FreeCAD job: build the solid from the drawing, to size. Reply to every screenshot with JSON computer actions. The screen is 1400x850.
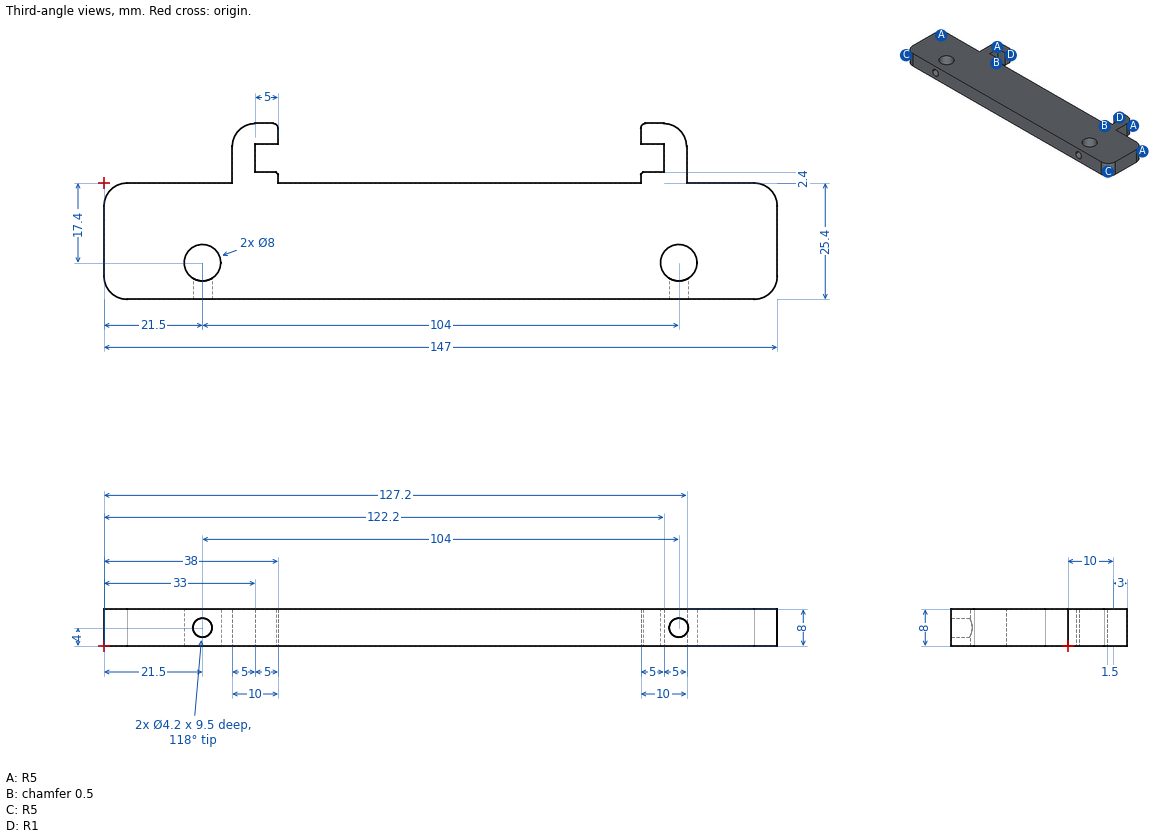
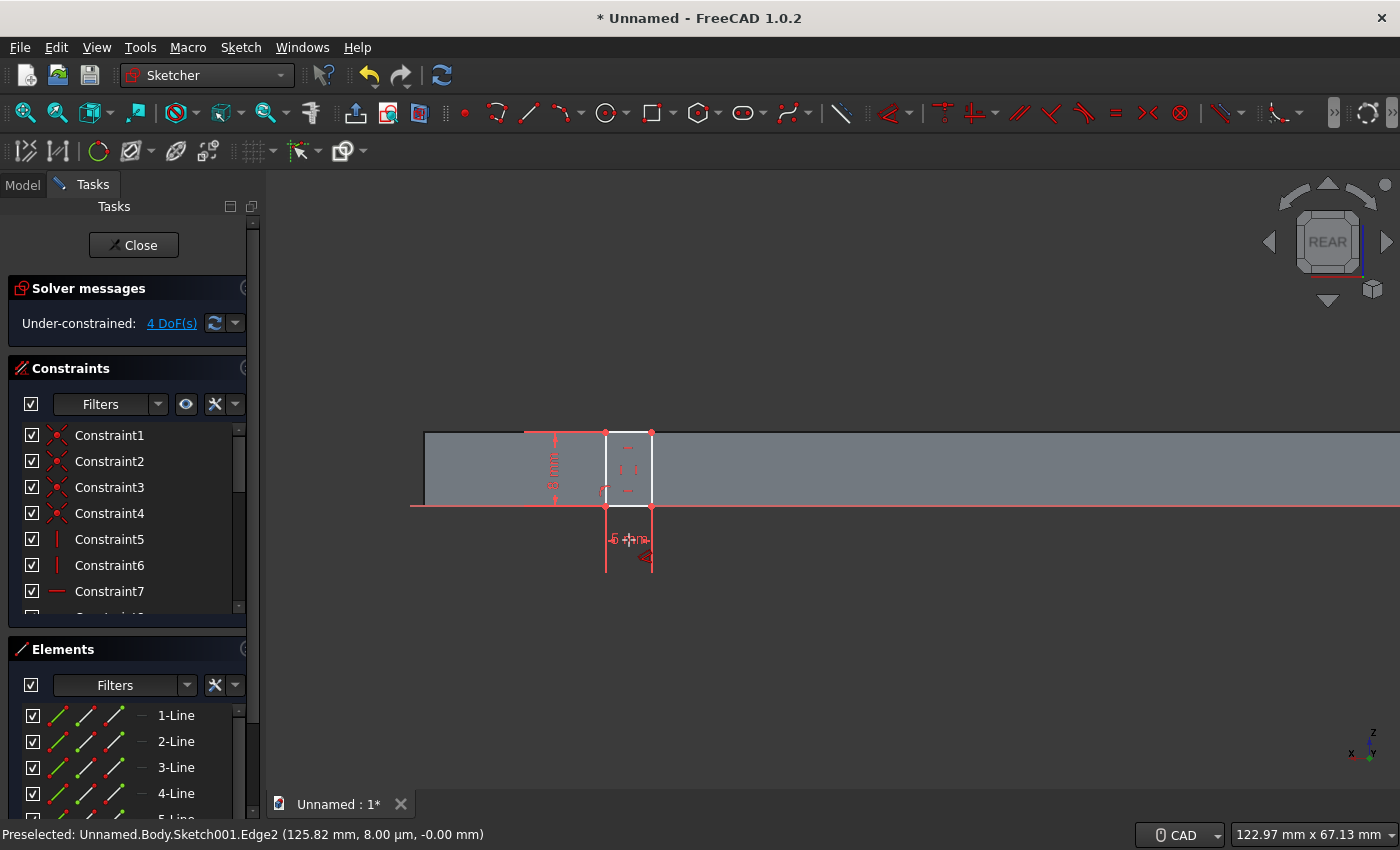
{"action": "scroll", "coordinate": [294, 492], "scroll_direction": "down", "scroll_amount": 3}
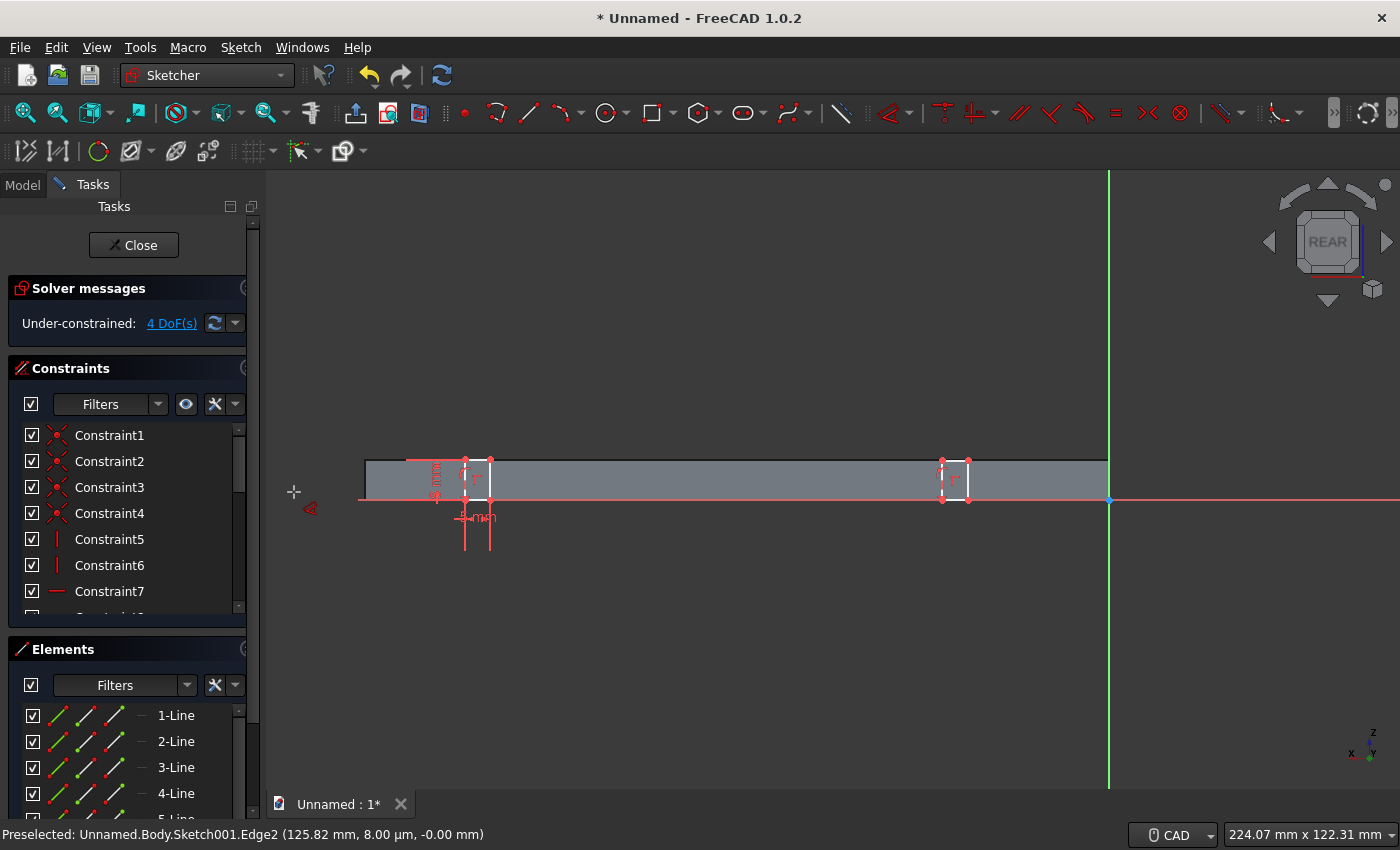
{"action": "left_click", "coordinate": [942, 473]}
{"action": "left_click", "coordinate": [908, 480]}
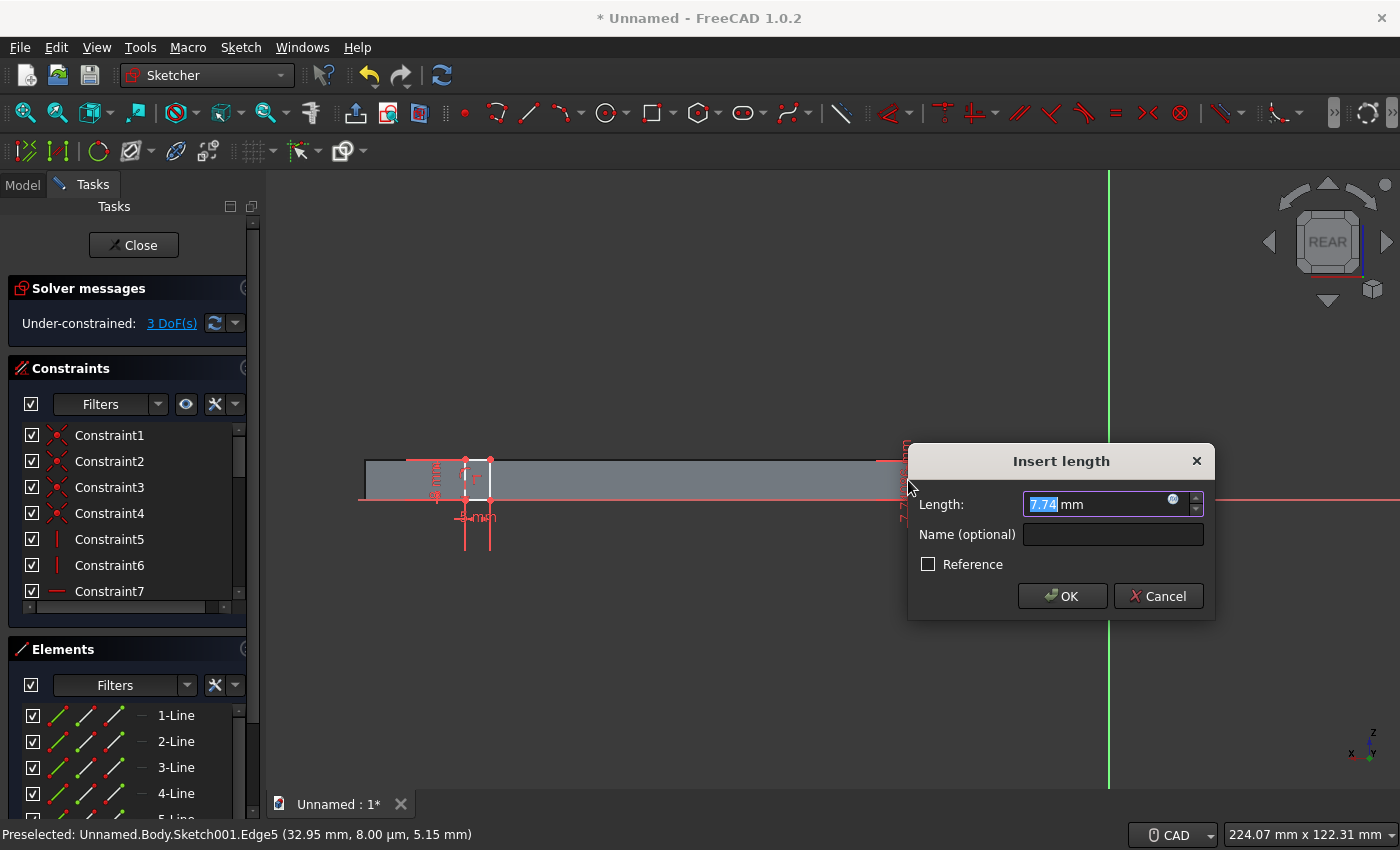
{"action": "type", "text": "8"}
{"action": "key", "text": "Return"}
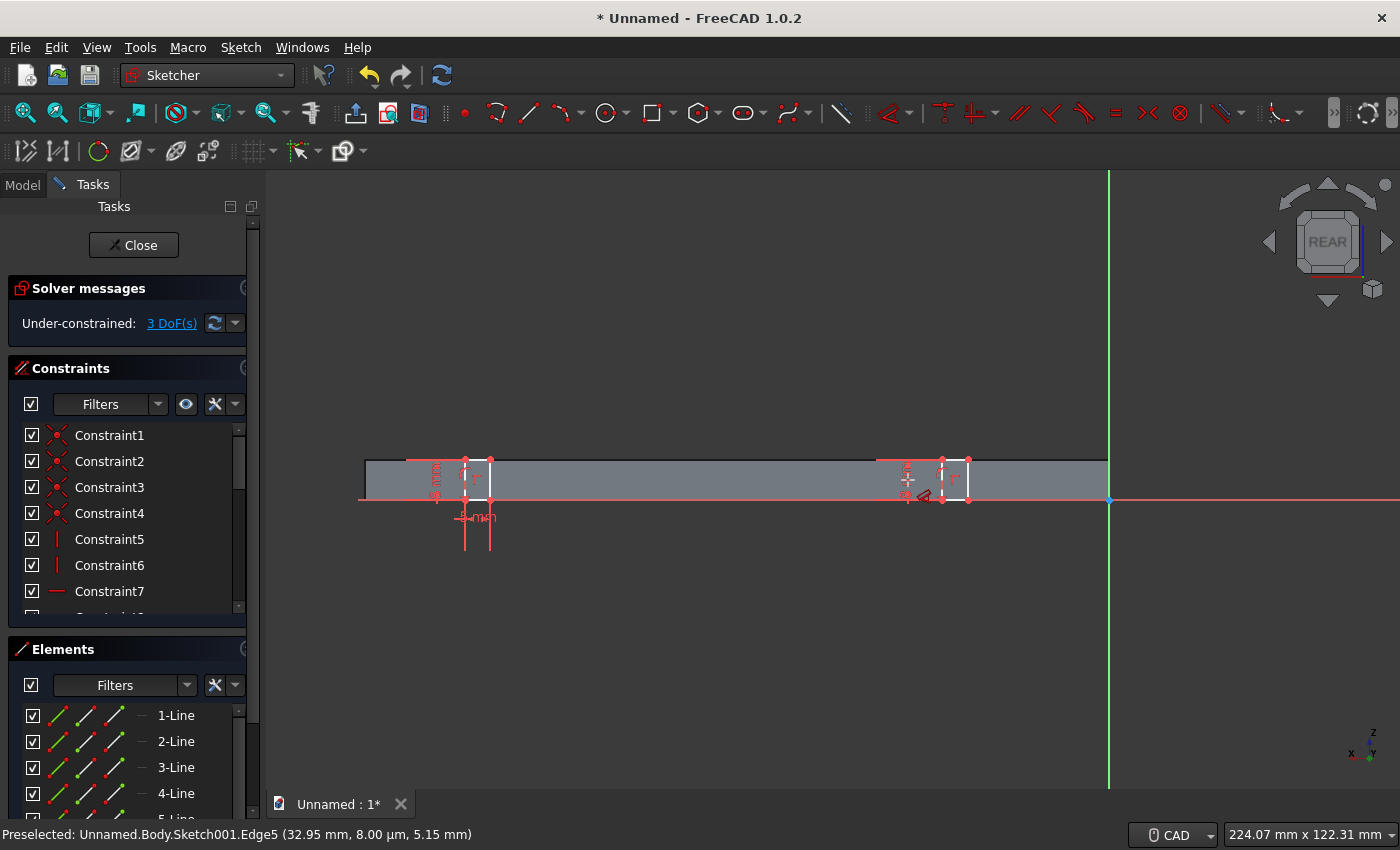
{"action": "scroll", "coordinate": [953, 500], "scroll_direction": "up", "scroll_amount": 3}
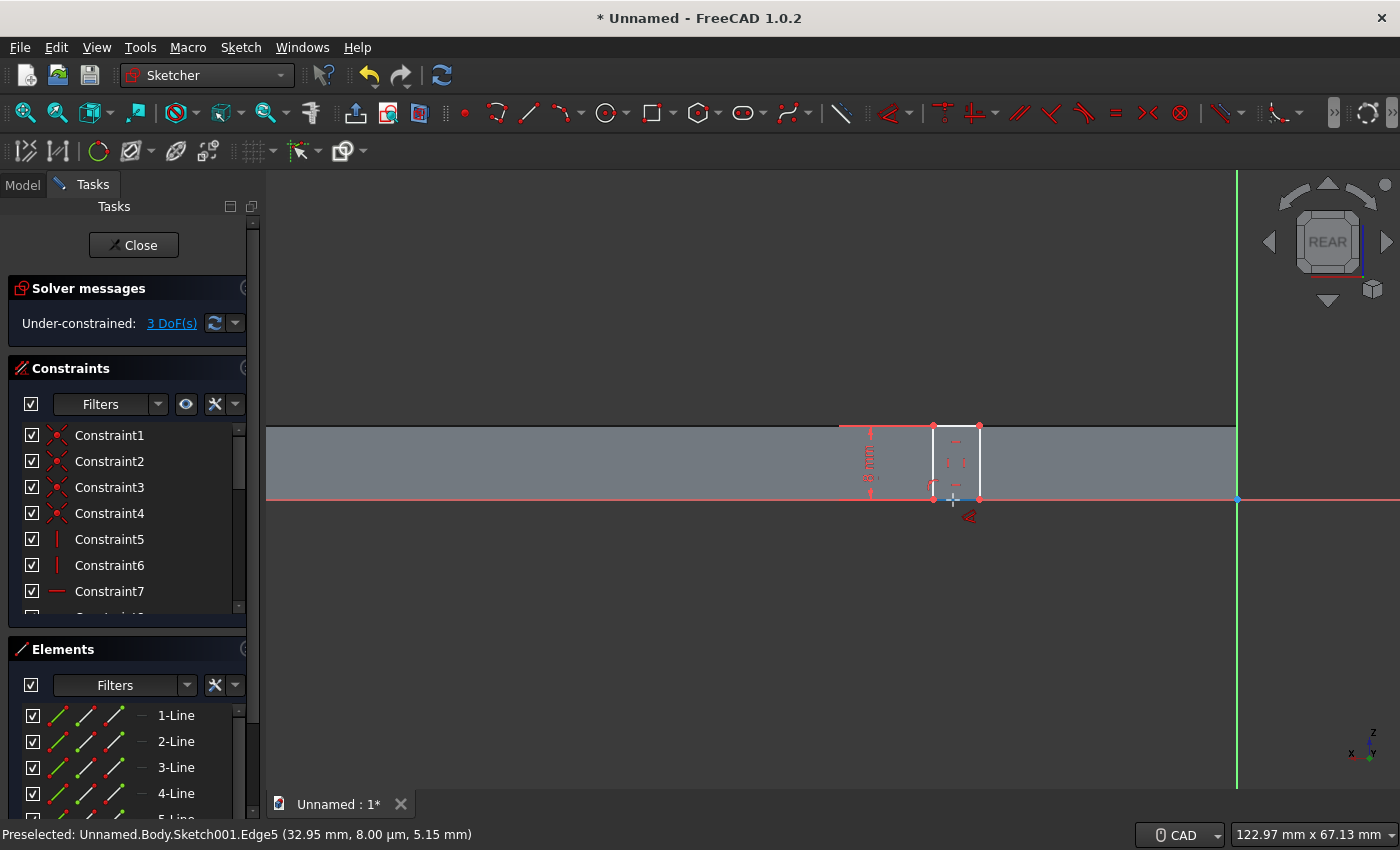
{"action": "left_click", "coordinate": [952, 500]}
{"action": "left_click", "coordinate": [956, 534]}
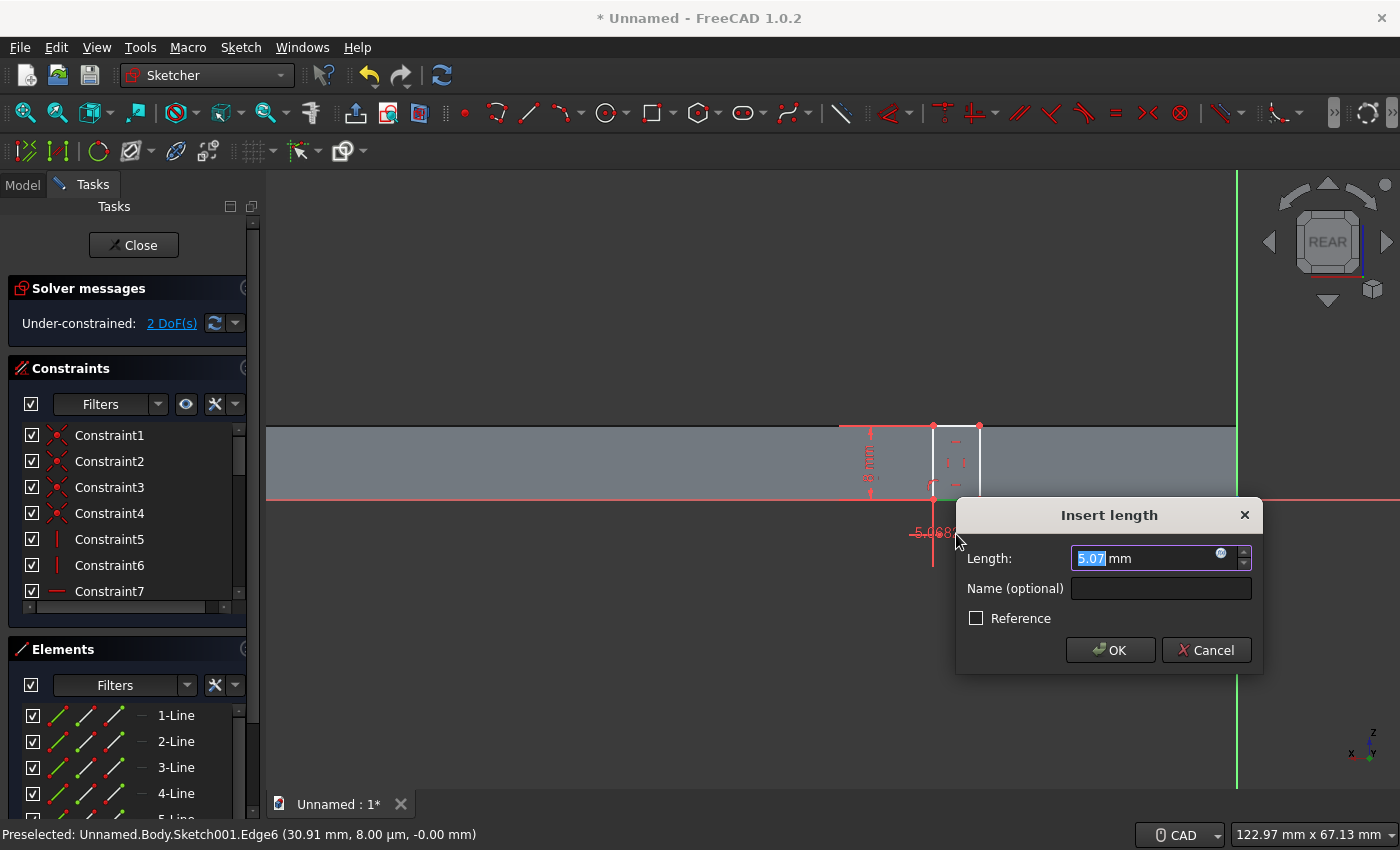
{"action": "type", "text": "5"}
{"action": "key", "text": "Return"}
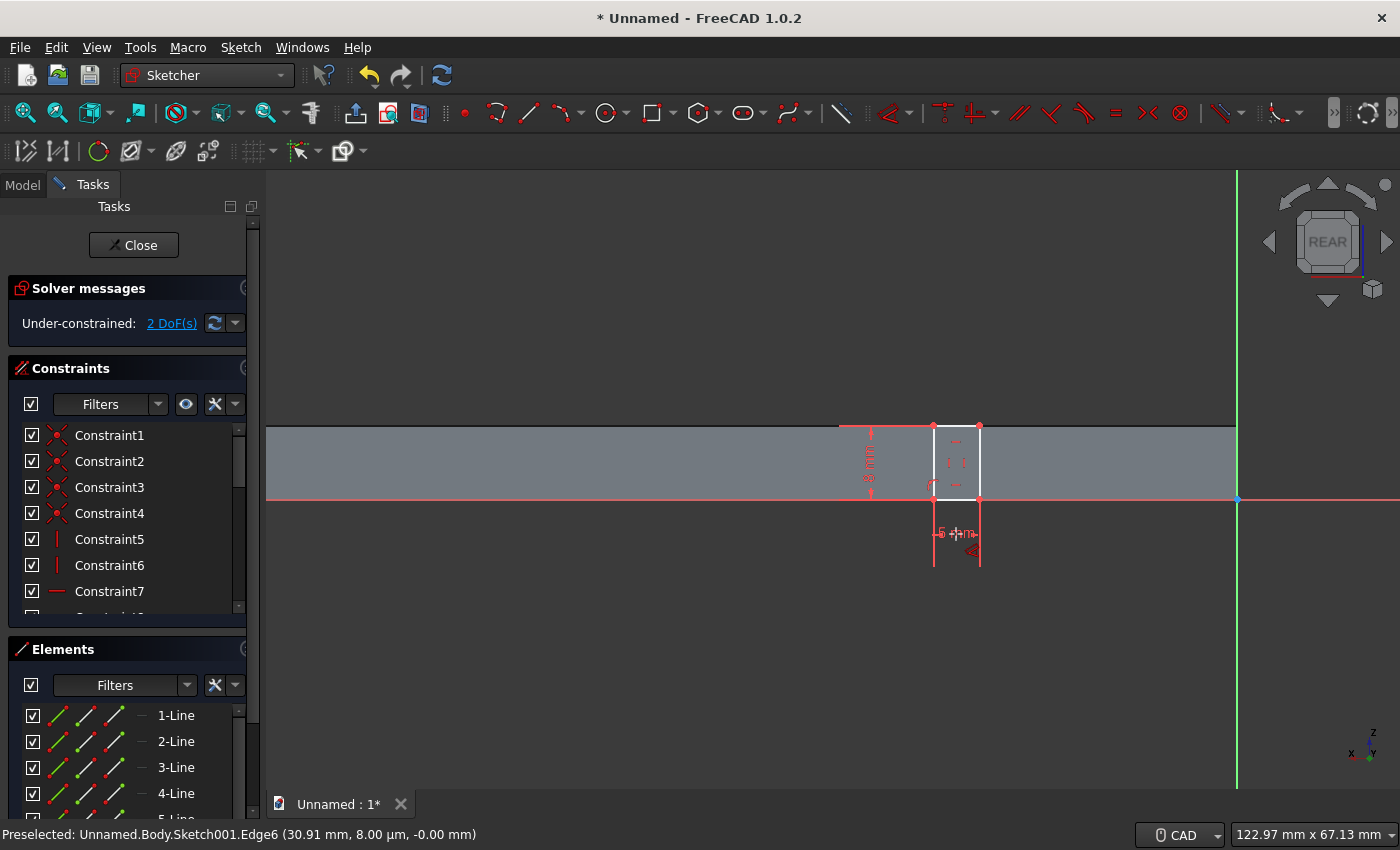
{"action": "left_click", "coordinate": [934, 426]}
{"action": "left_click", "coordinate": [1084, 534]}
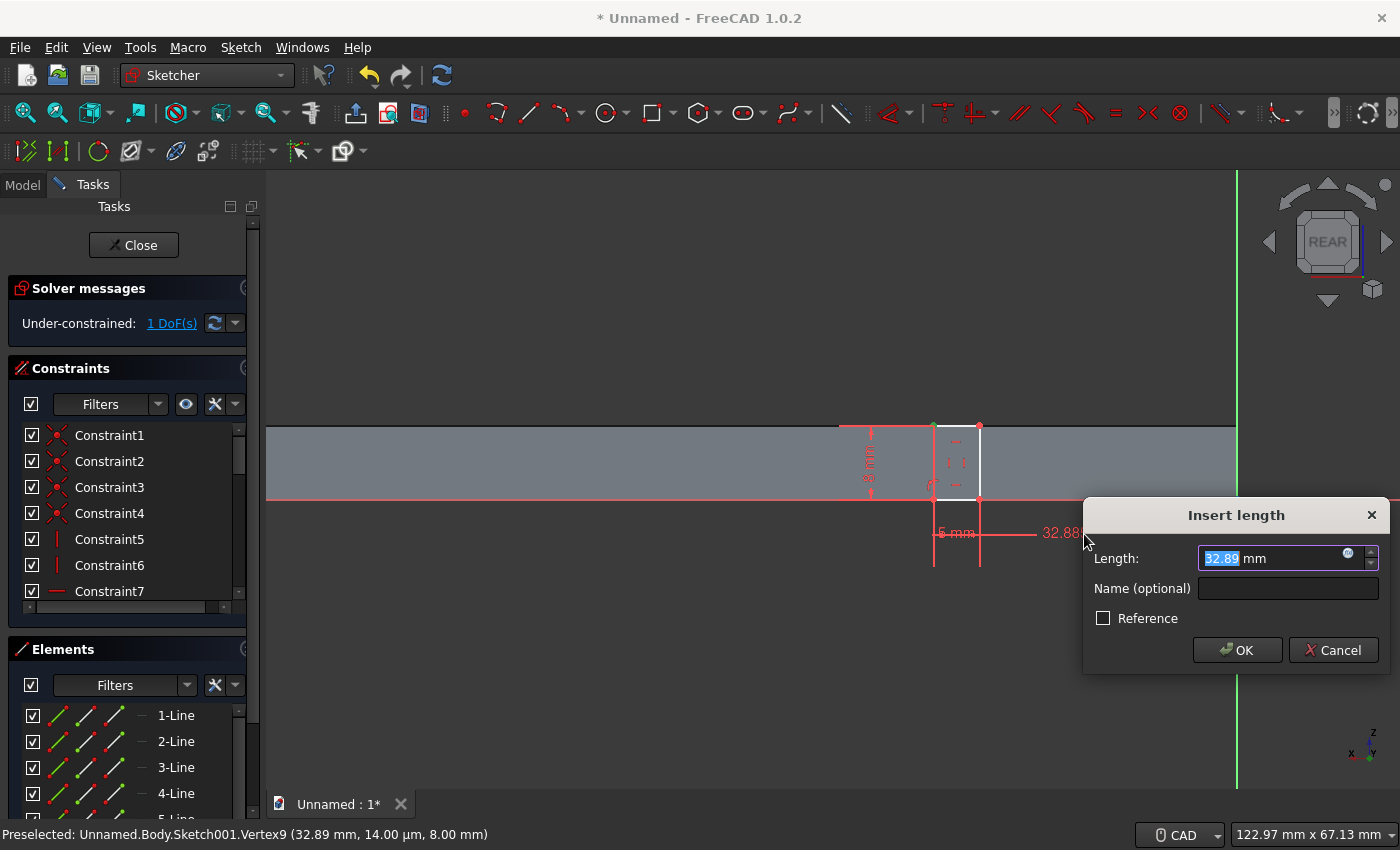
{"action": "type", "text": "33"}
{"action": "key", "text": "Return"}